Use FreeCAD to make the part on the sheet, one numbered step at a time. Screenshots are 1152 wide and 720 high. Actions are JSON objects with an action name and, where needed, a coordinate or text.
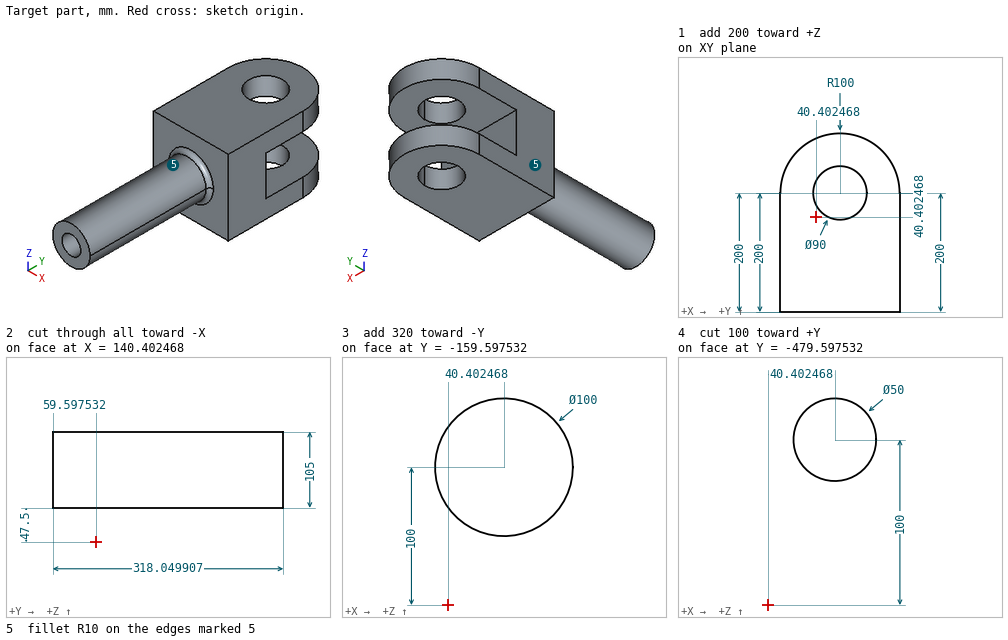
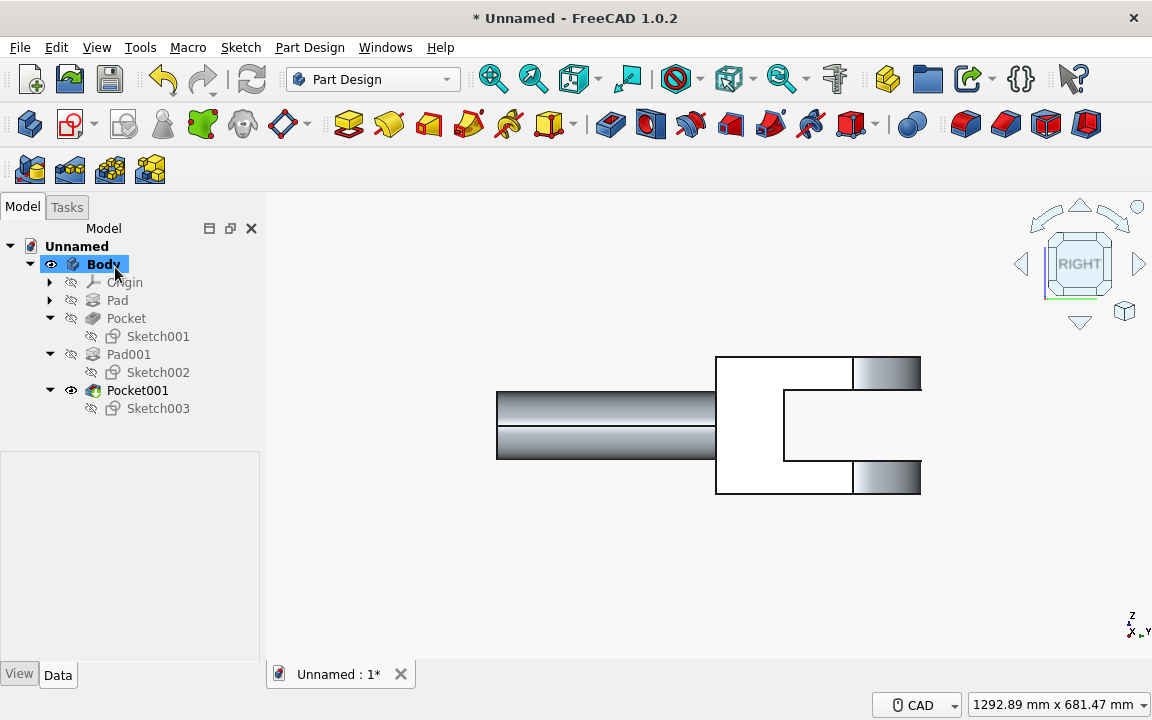
{"action": "key", "text": "5"}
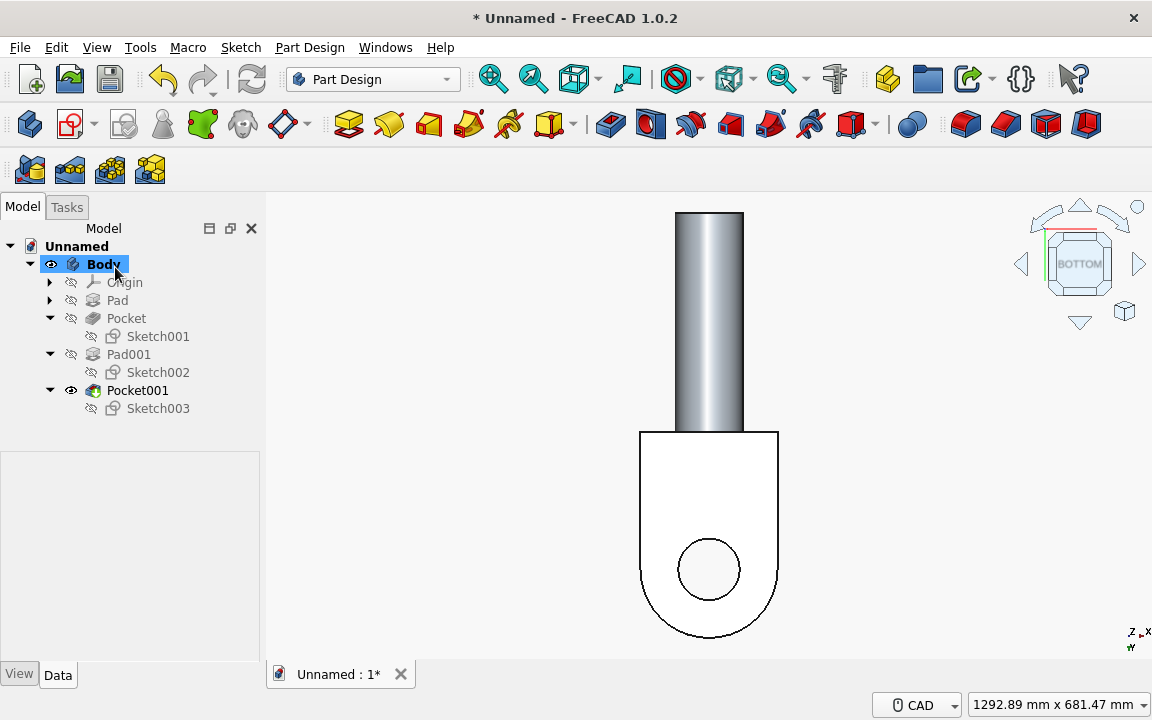
{"action": "key", "text": "4"}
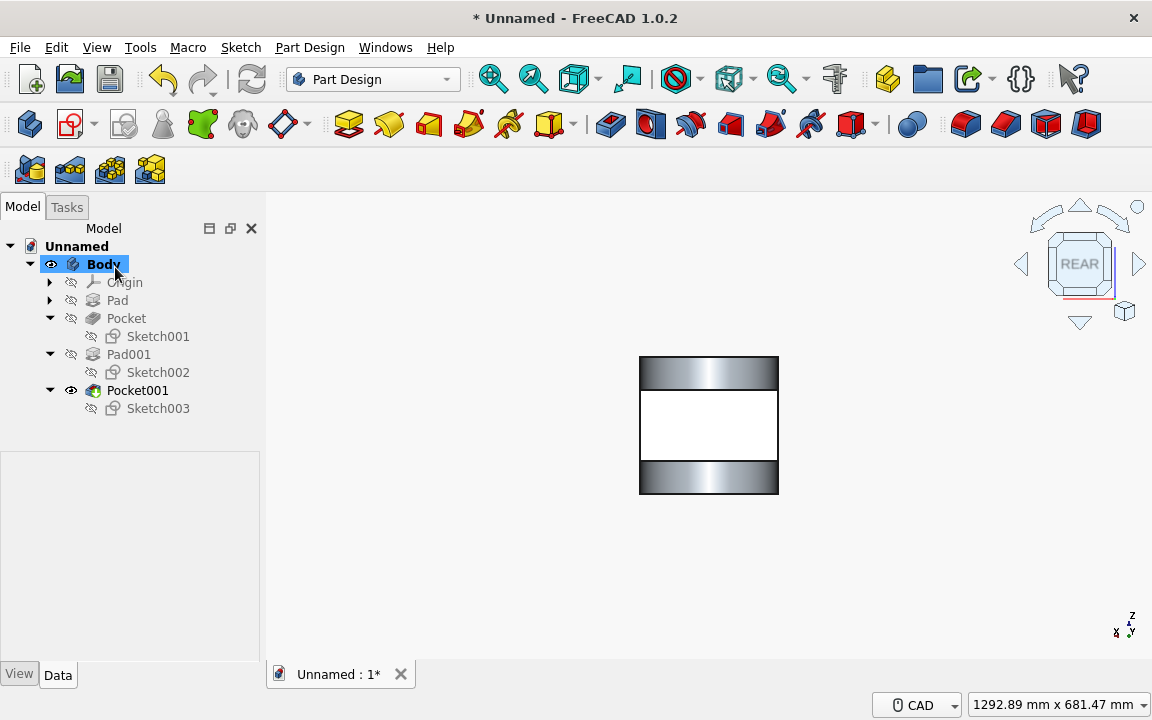
{"action": "key", "text": "v f"}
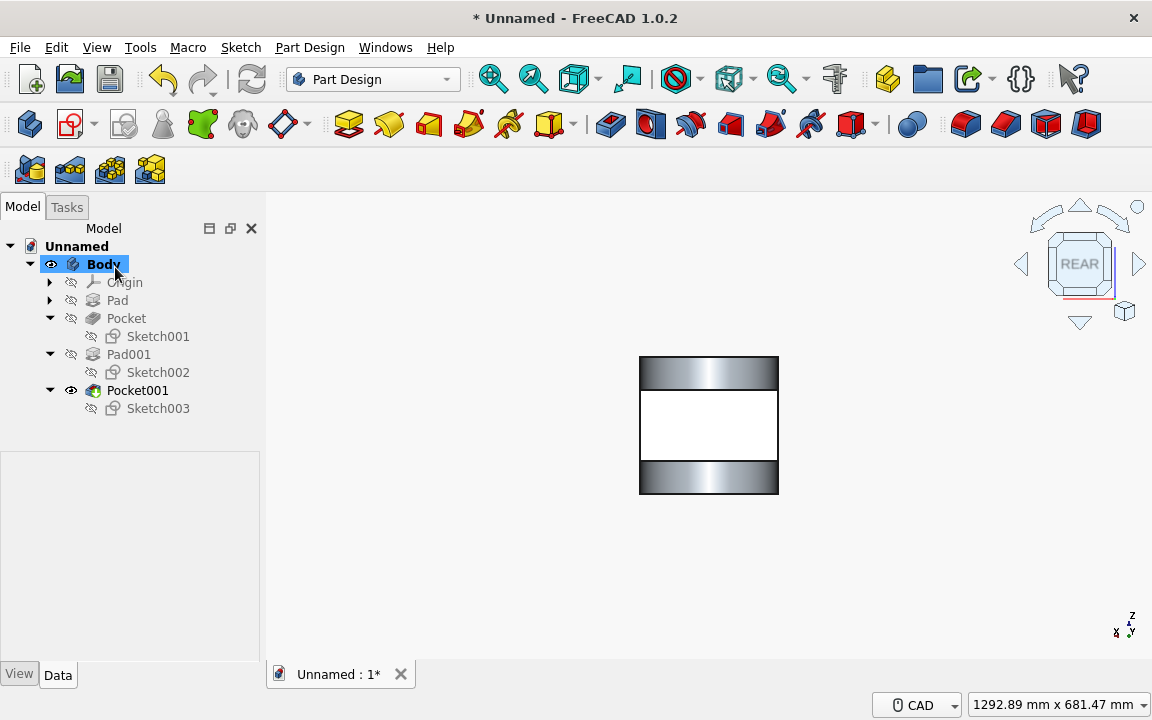
{"action": "key", "text": "6"}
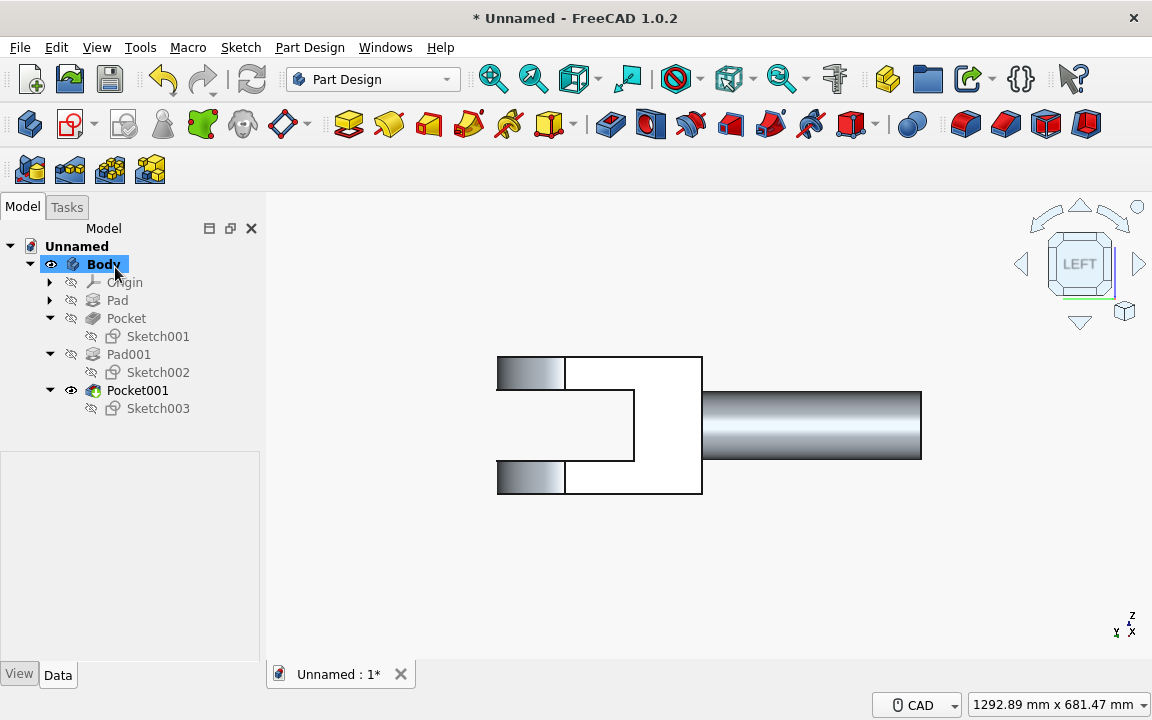
{"action": "key", "text": "v 3"}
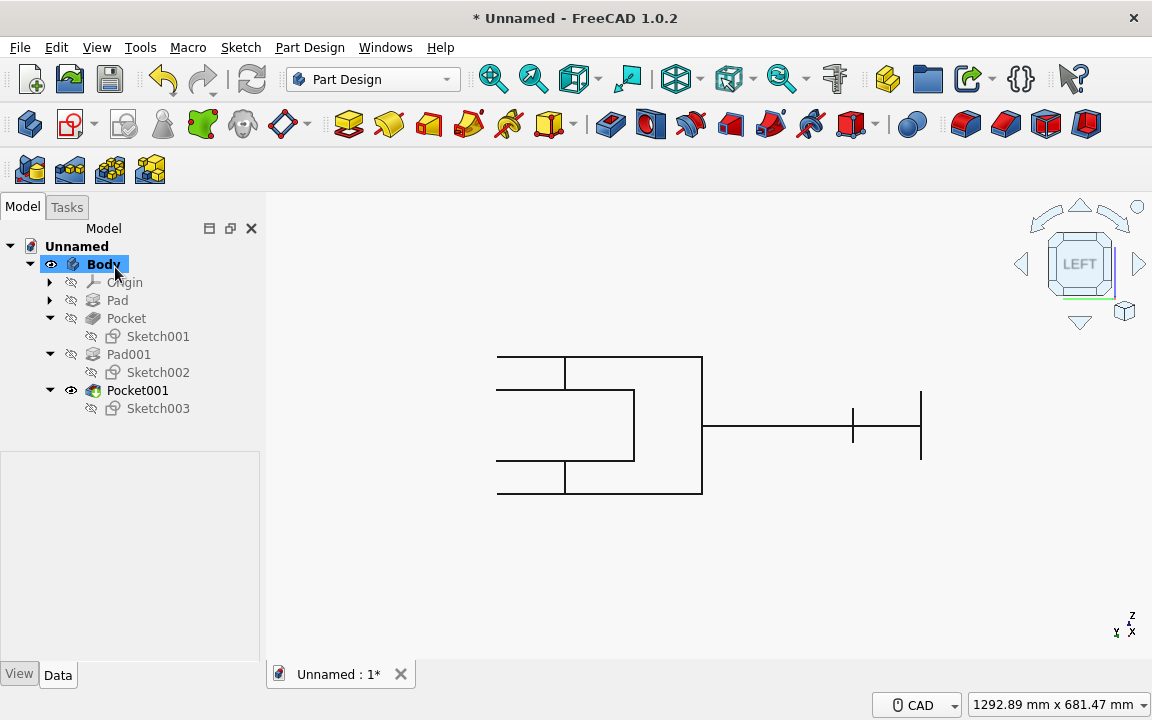
{"action": "key", "text": "0"}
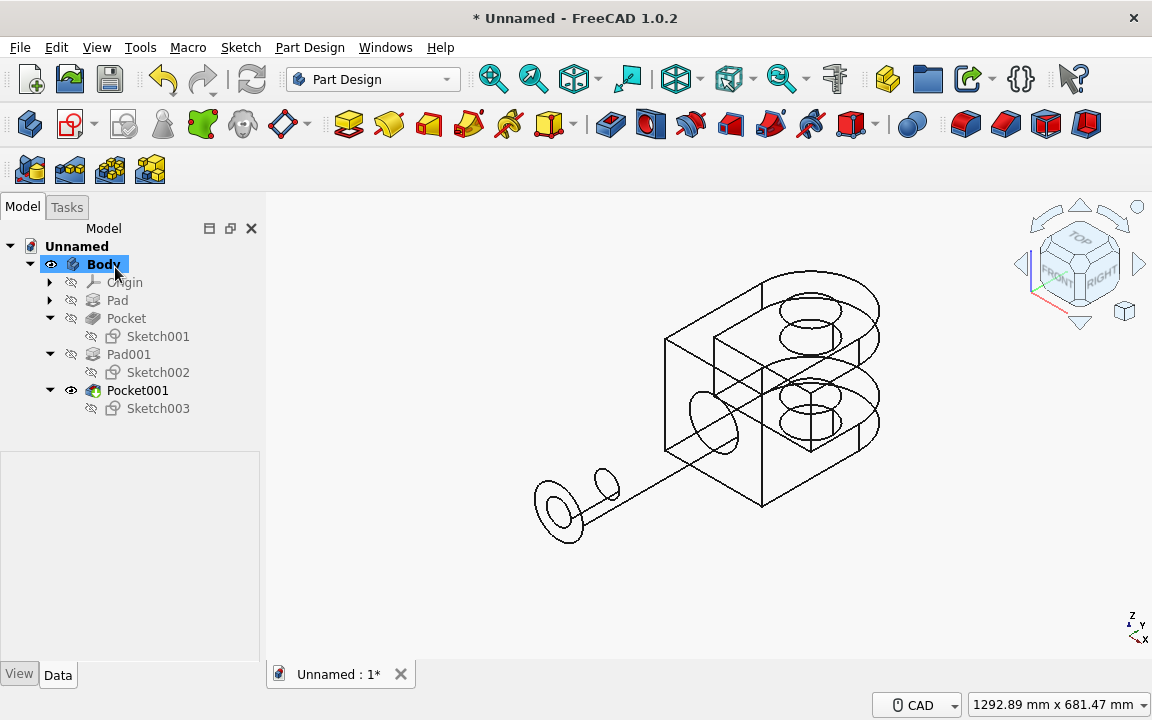
{"action": "left_click", "coordinate": [690, 408]}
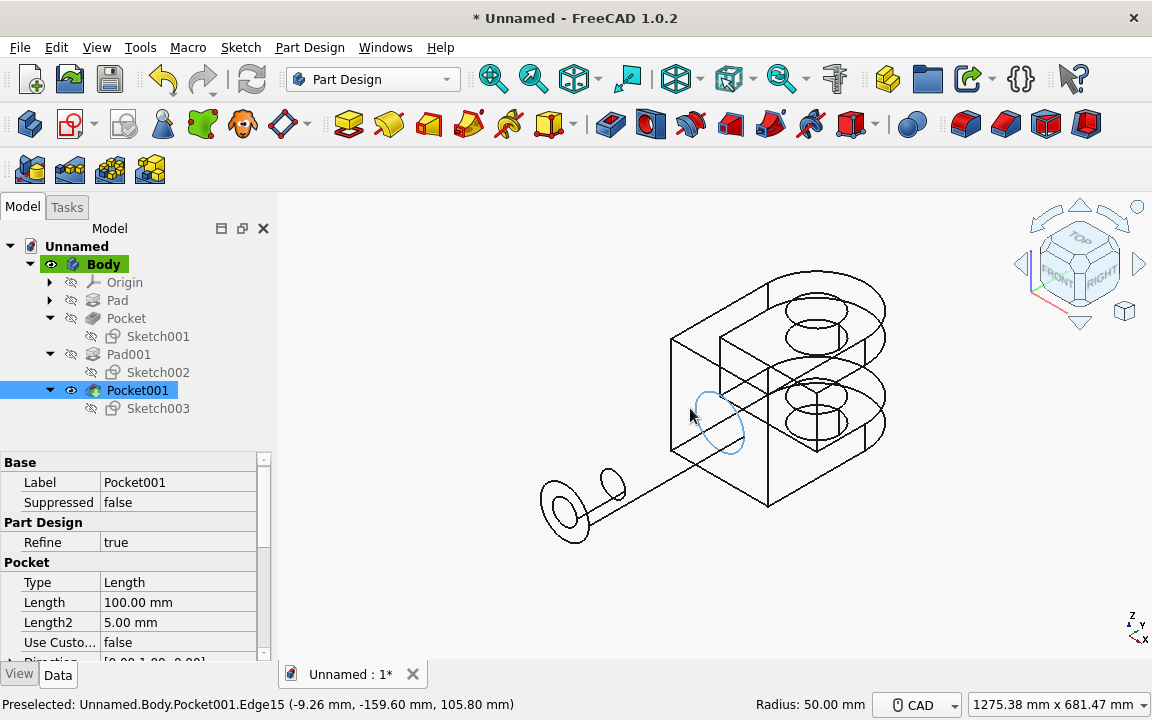
{"action": "key", "text": "v 1"}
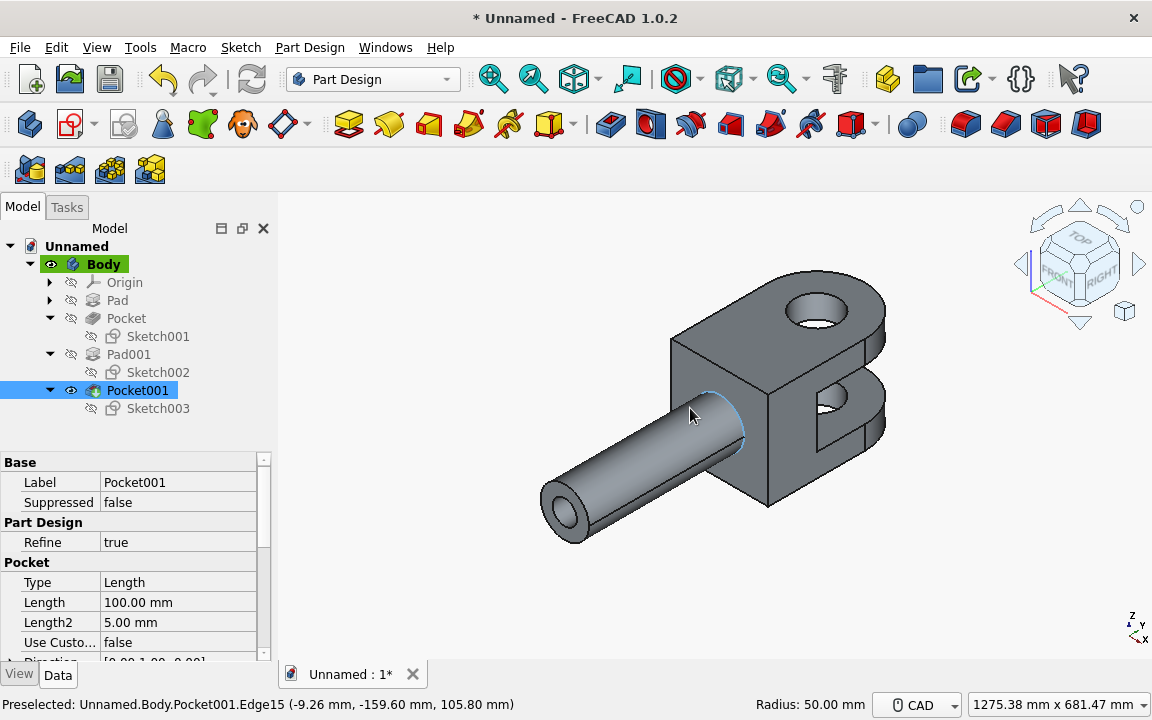
{"action": "left_click", "coordinate": [966, 124]}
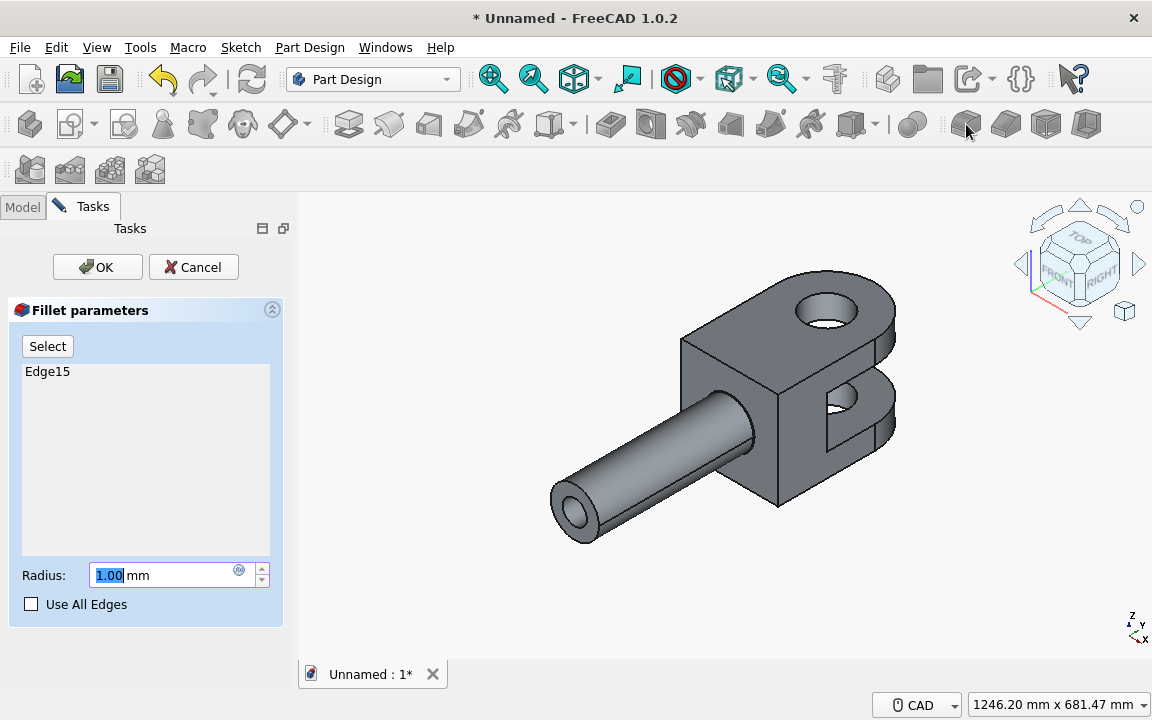
{"action": "type", "text": "10"}
{"action": "key", "text": "Tab"}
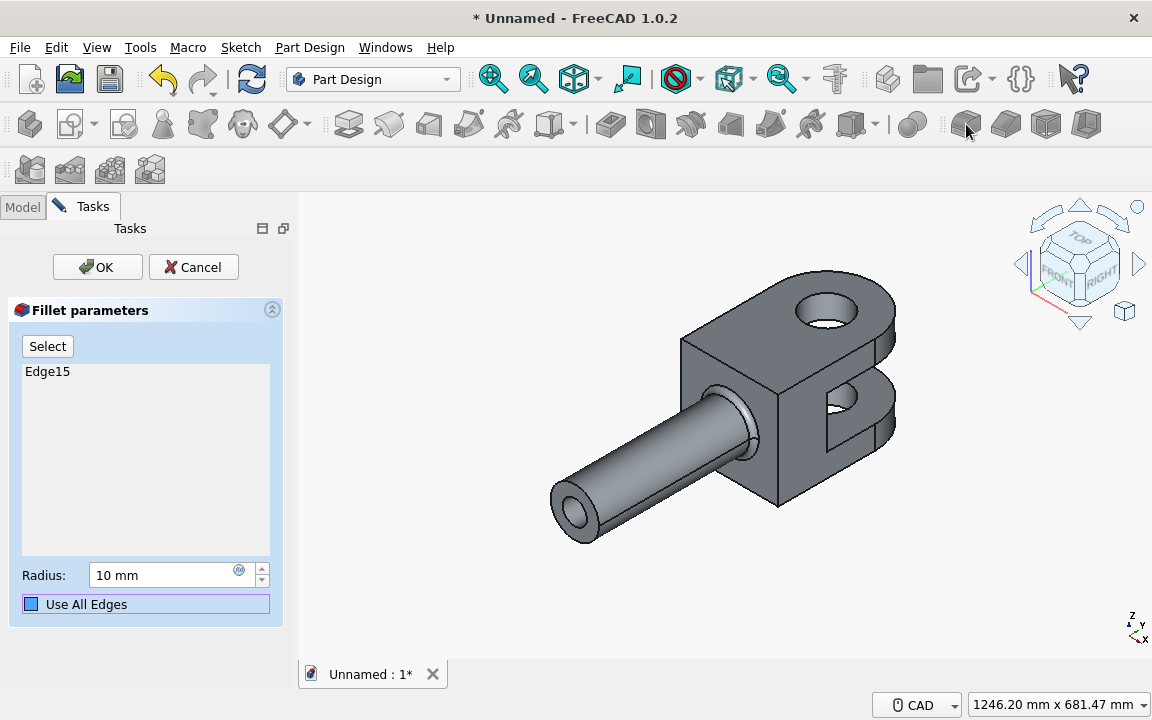
{"action": "left_click", "coordinate": [98, 267]}